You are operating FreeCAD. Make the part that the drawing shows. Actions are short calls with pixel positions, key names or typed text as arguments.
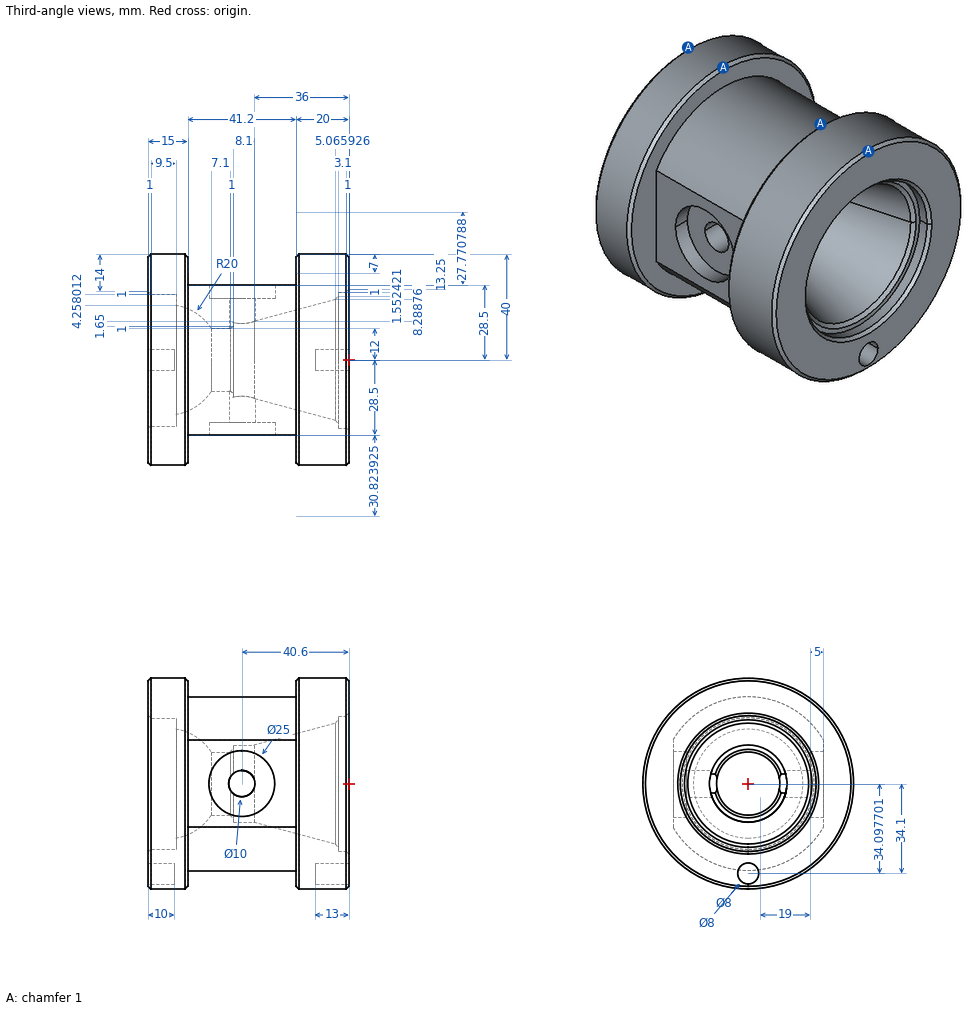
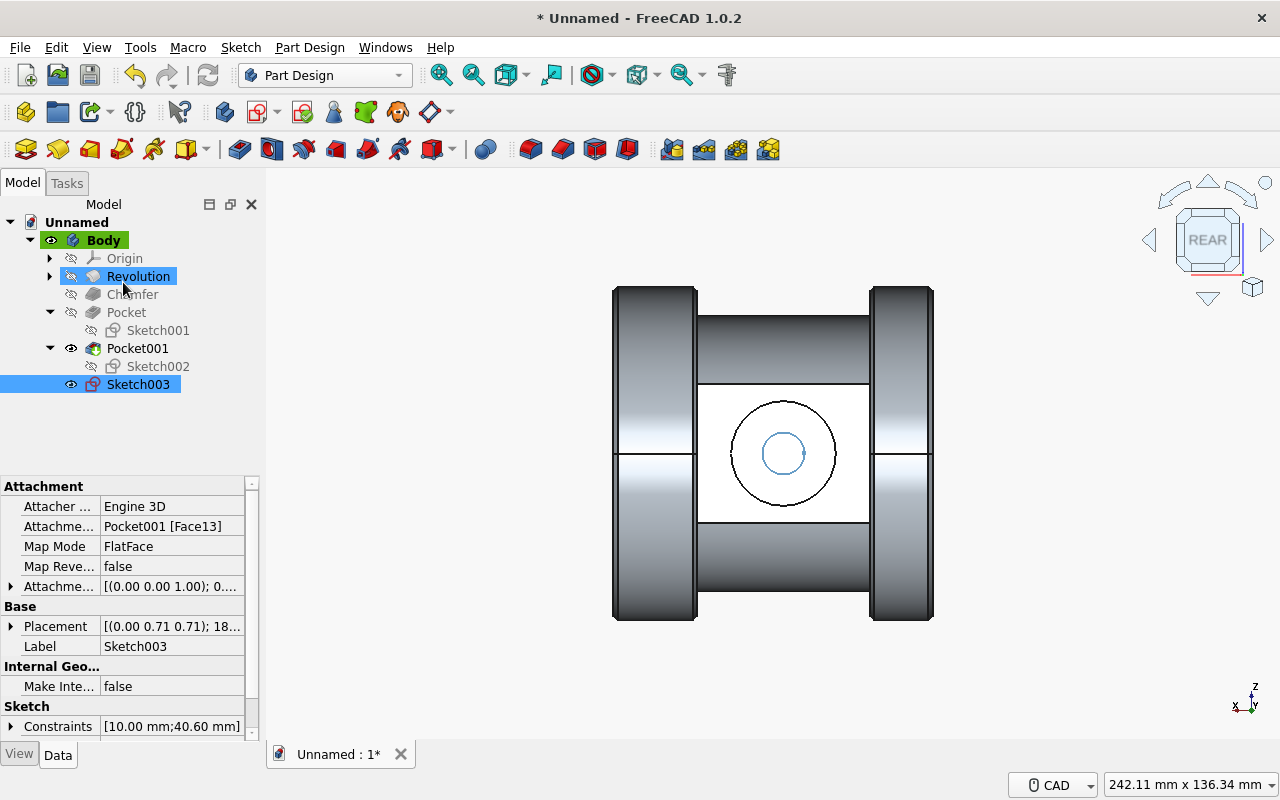
click(240, 150)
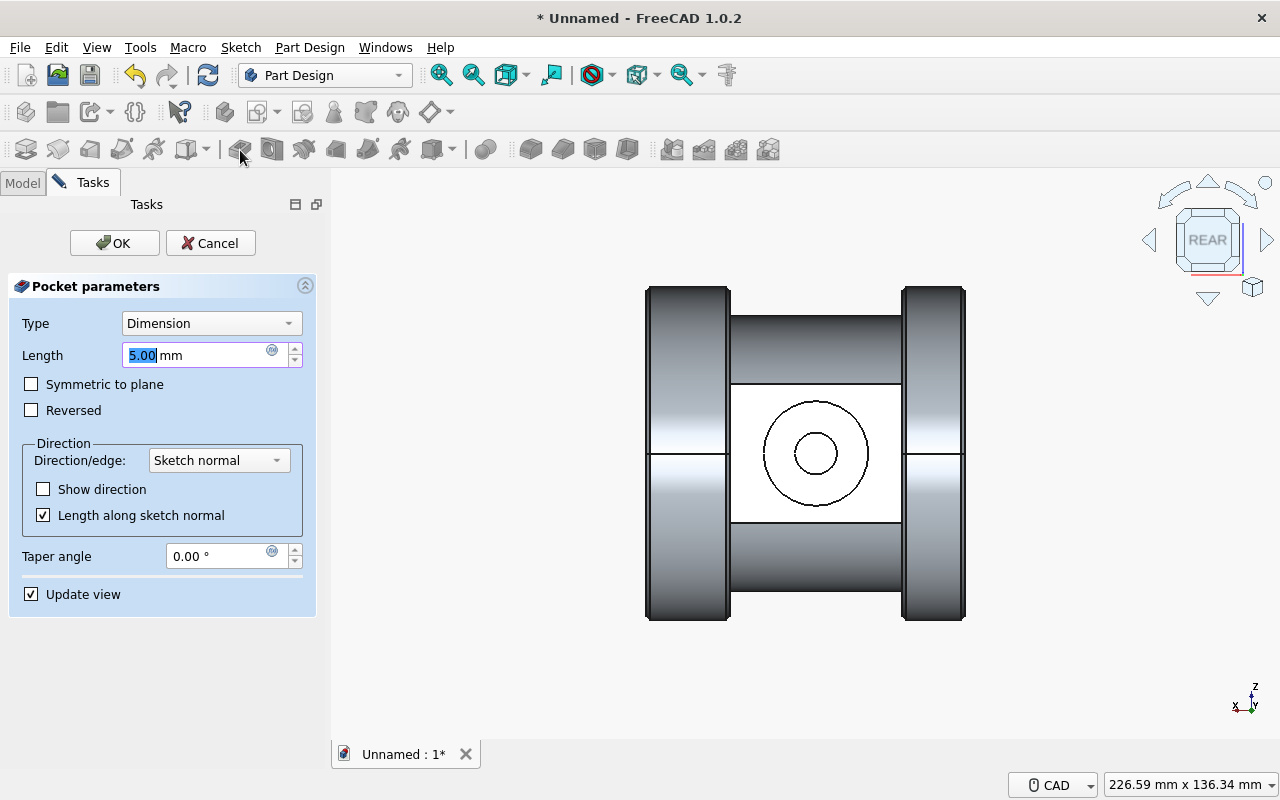
text(19)
key(Tab)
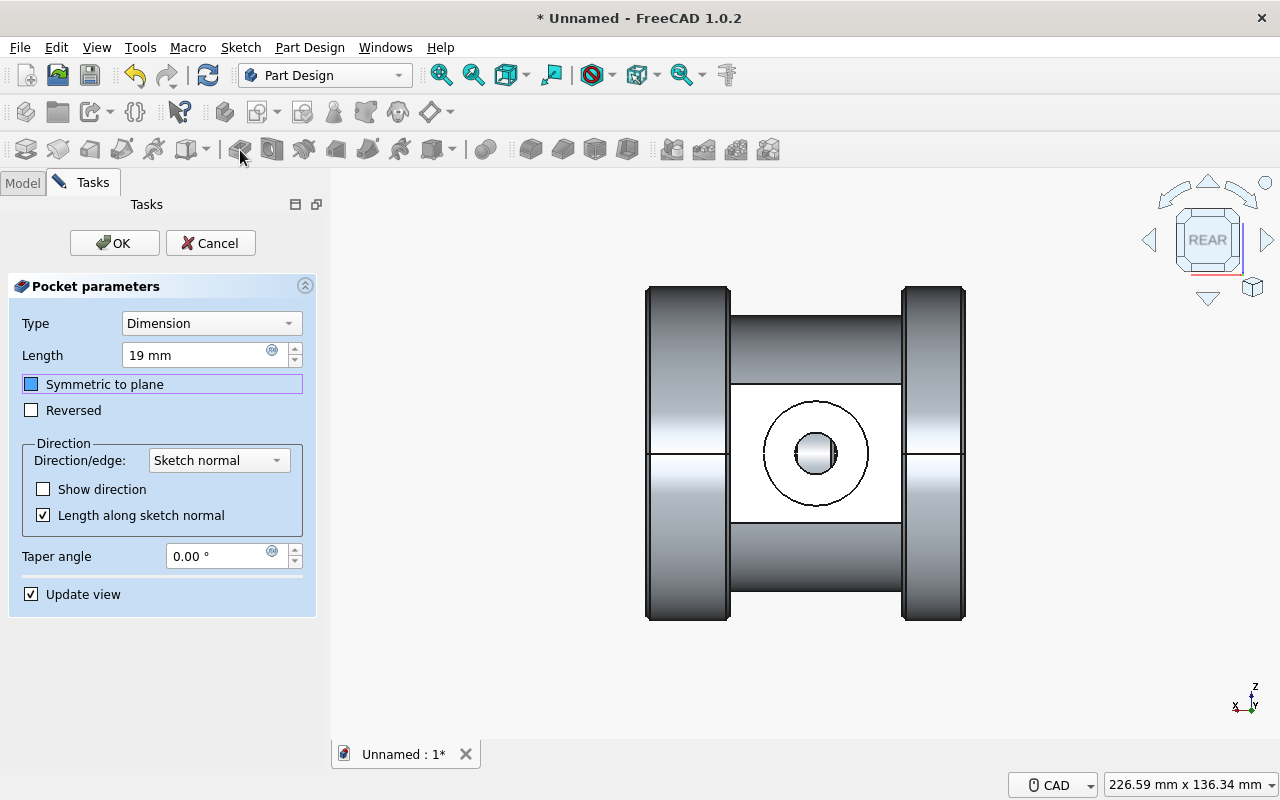
click(115, 243)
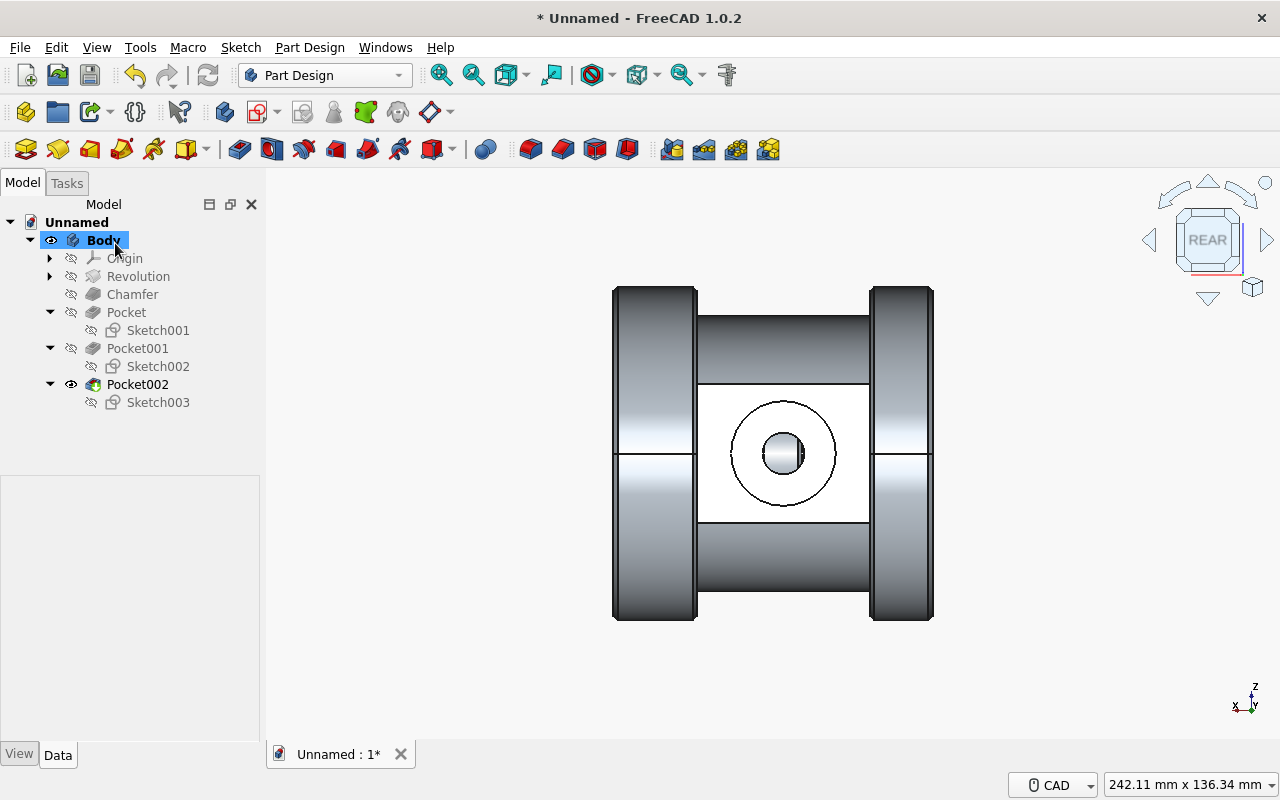
click(116, 348)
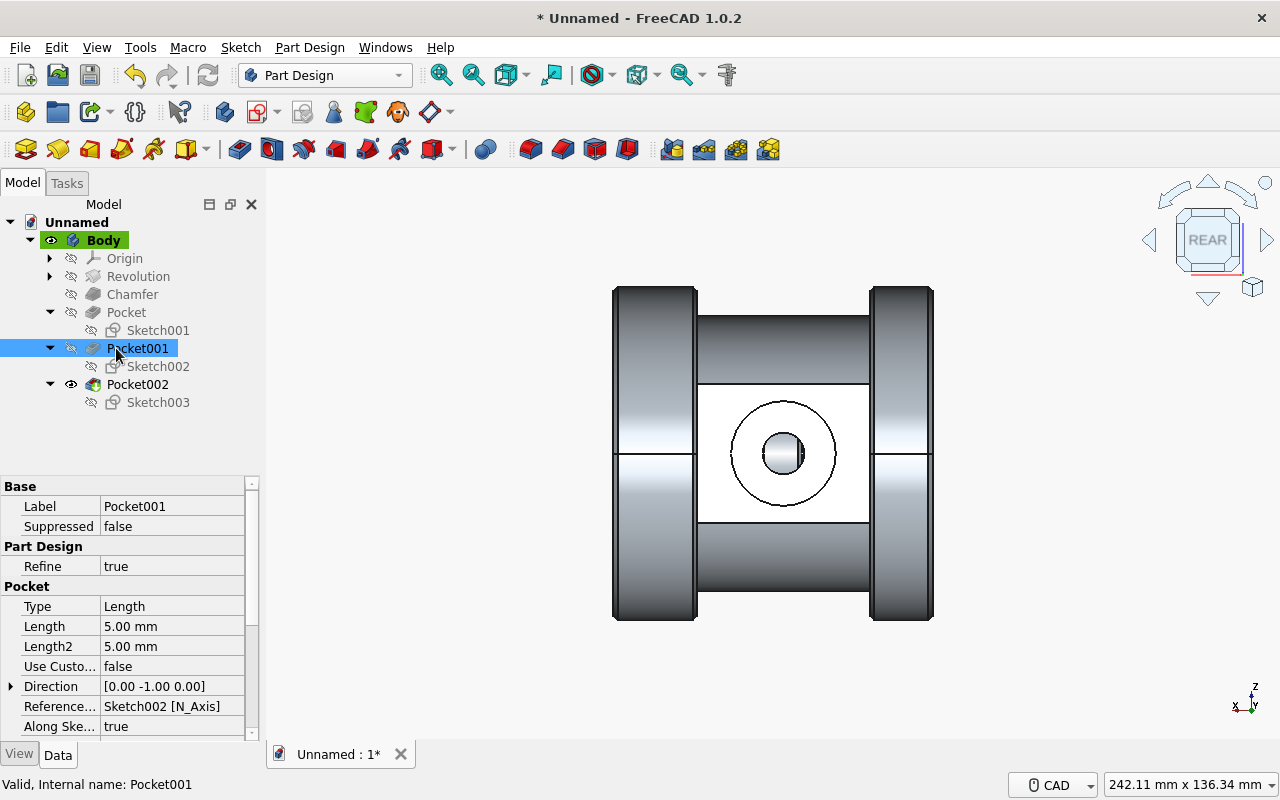
click(116, 384, ctrl)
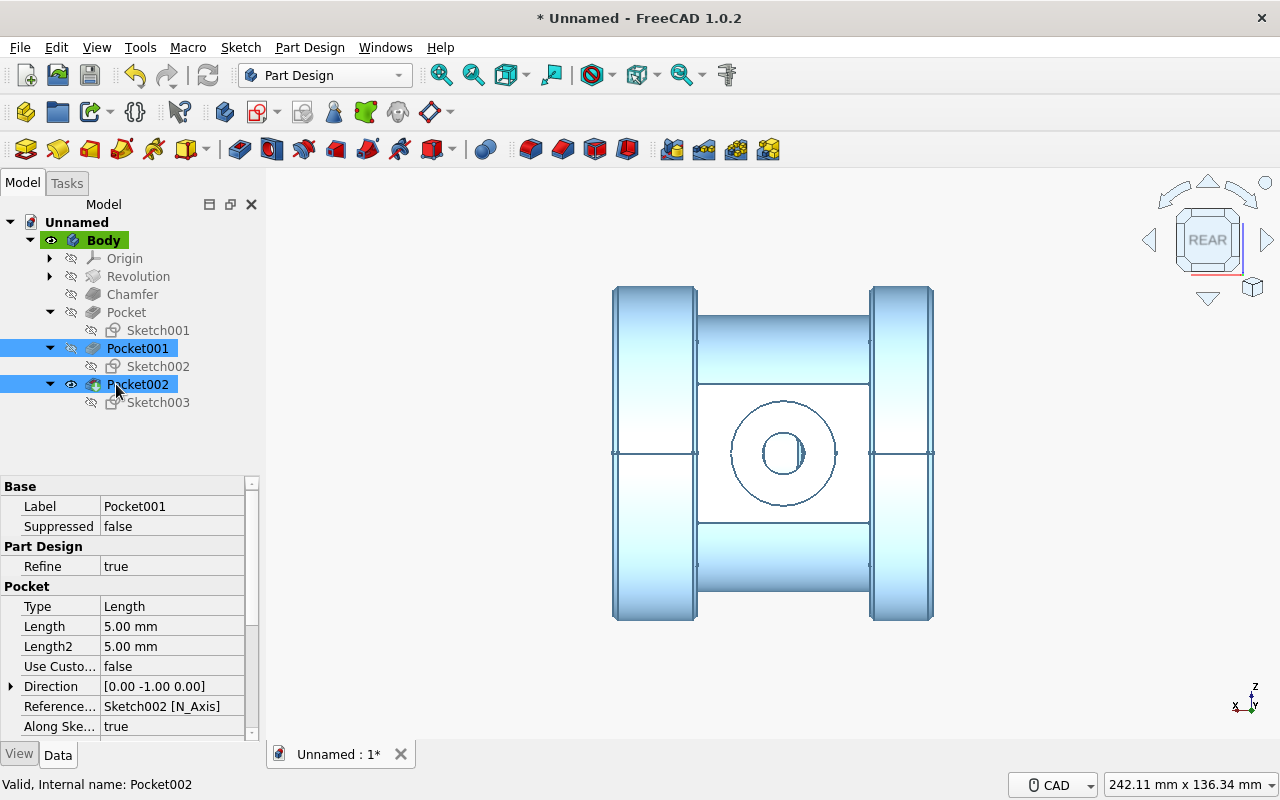
click(672, 150)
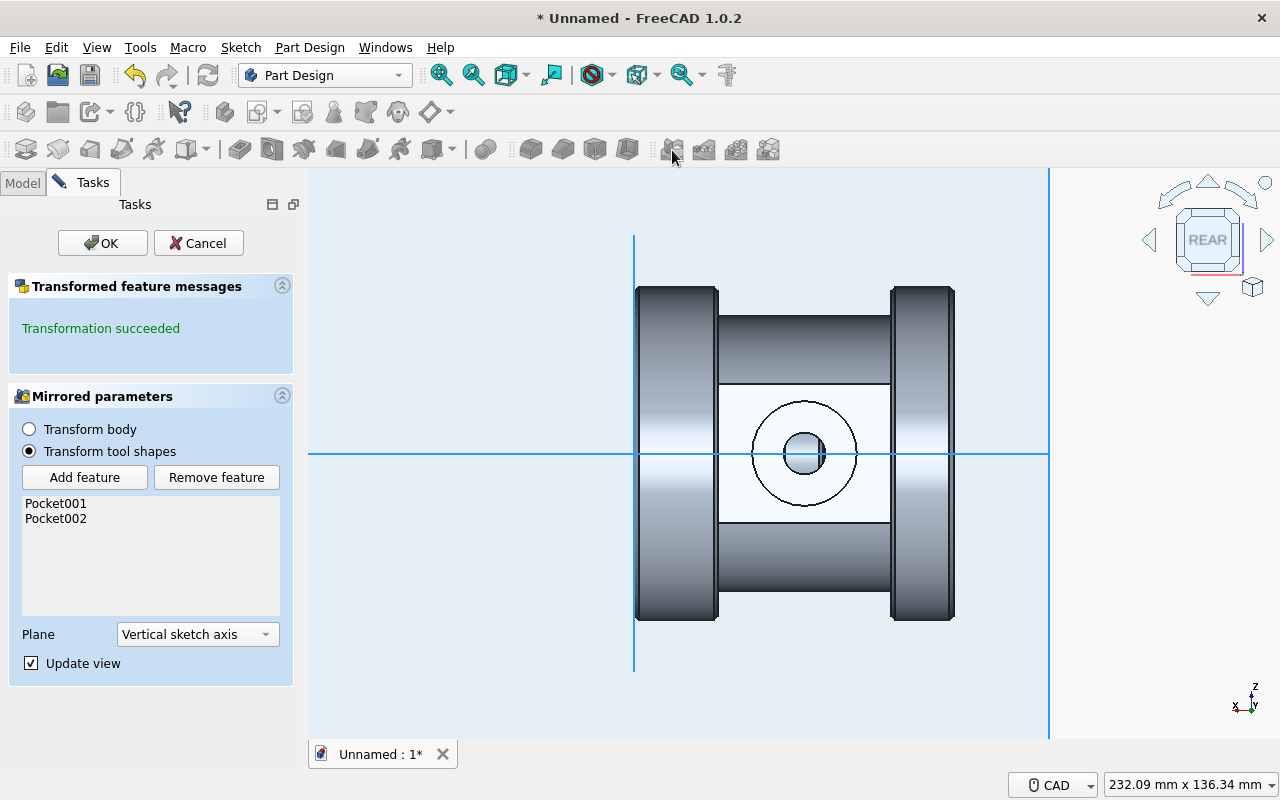
click(198, 634)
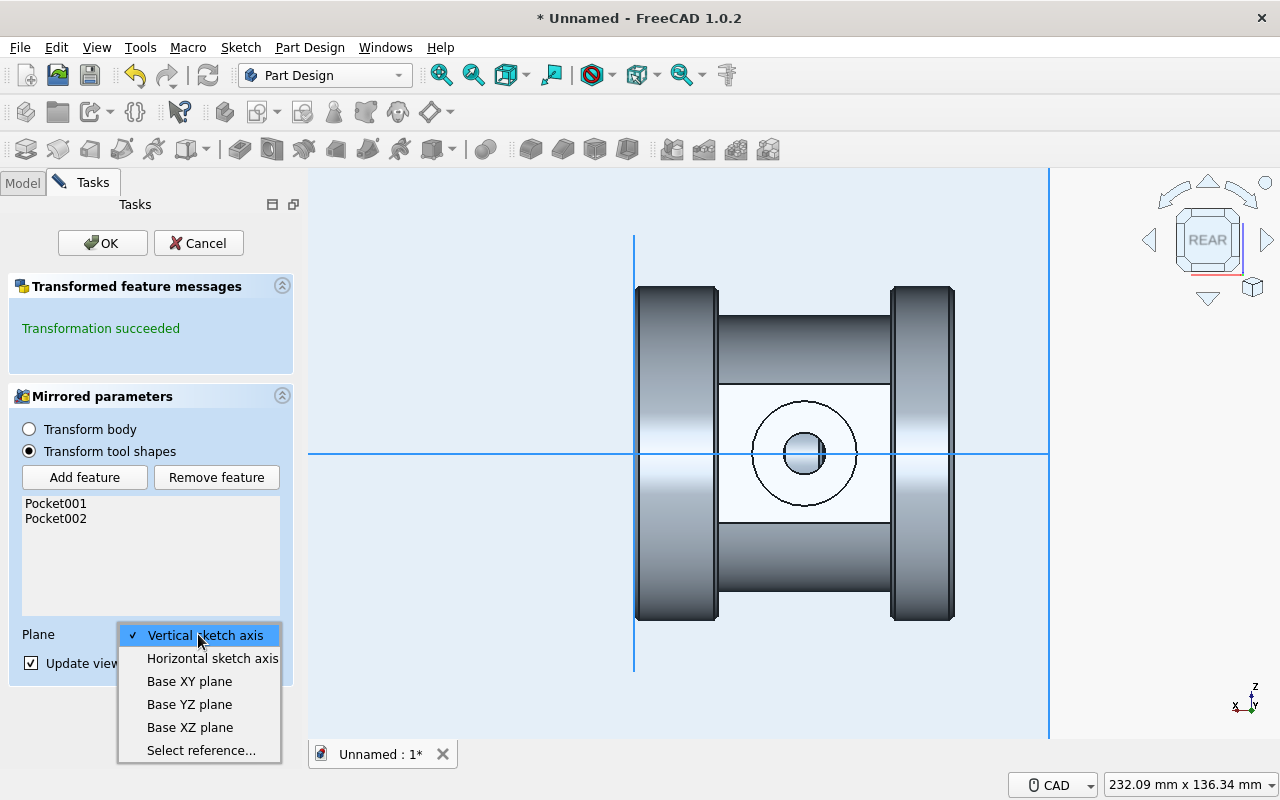
click(198, 728)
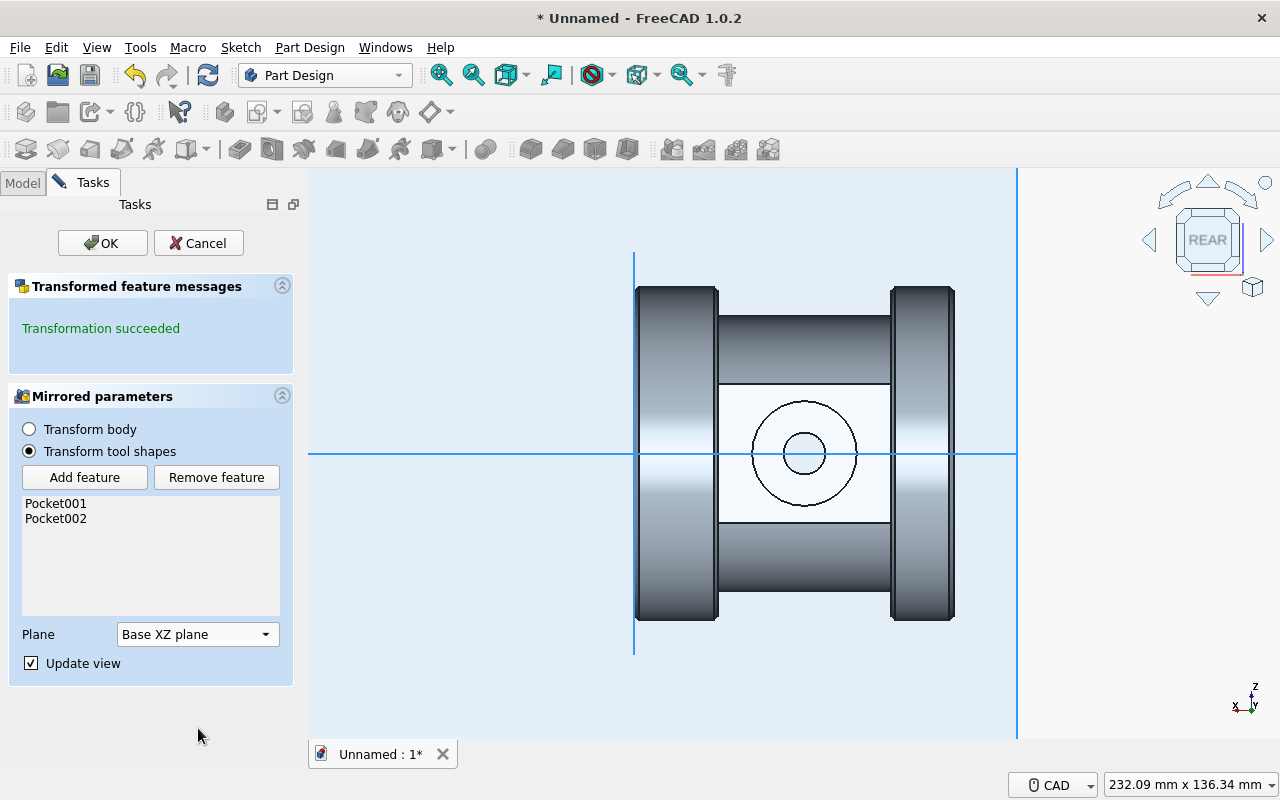
click(103, 243)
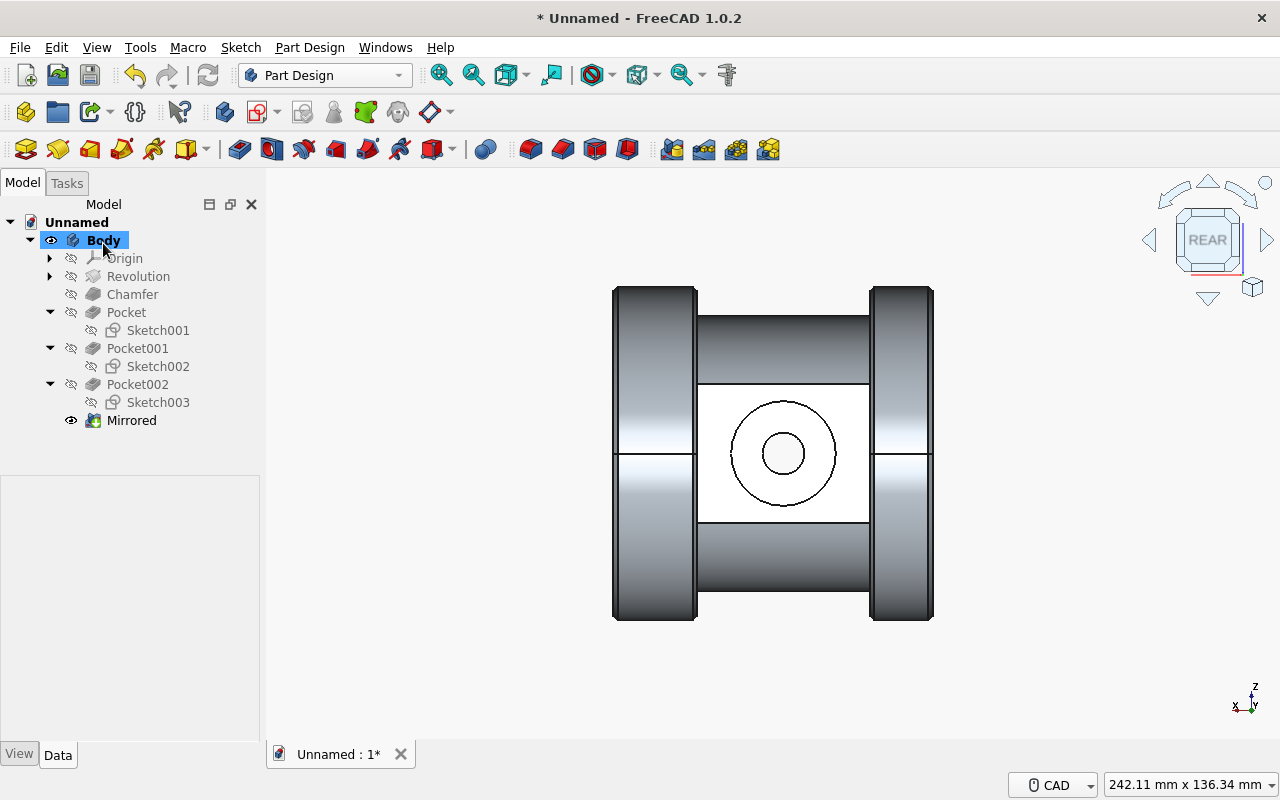
key(6)